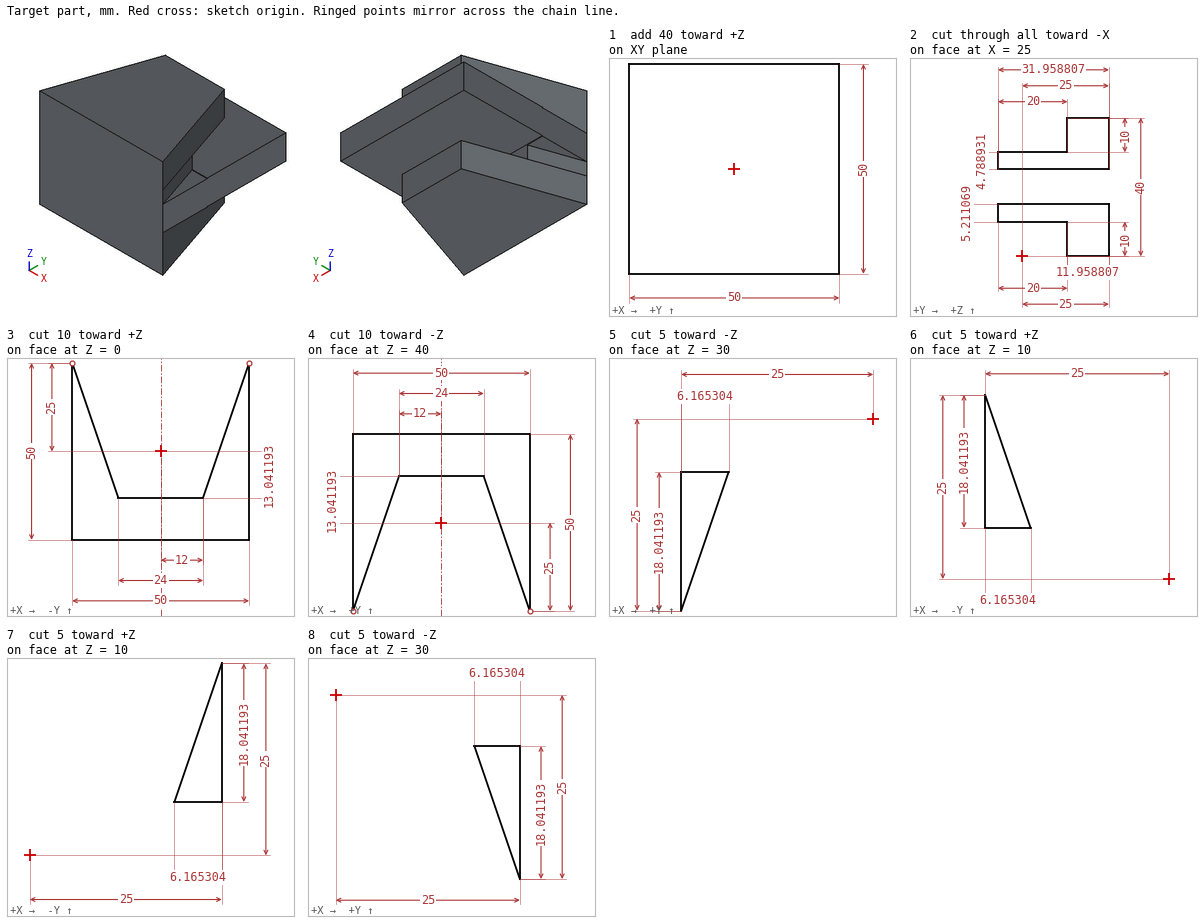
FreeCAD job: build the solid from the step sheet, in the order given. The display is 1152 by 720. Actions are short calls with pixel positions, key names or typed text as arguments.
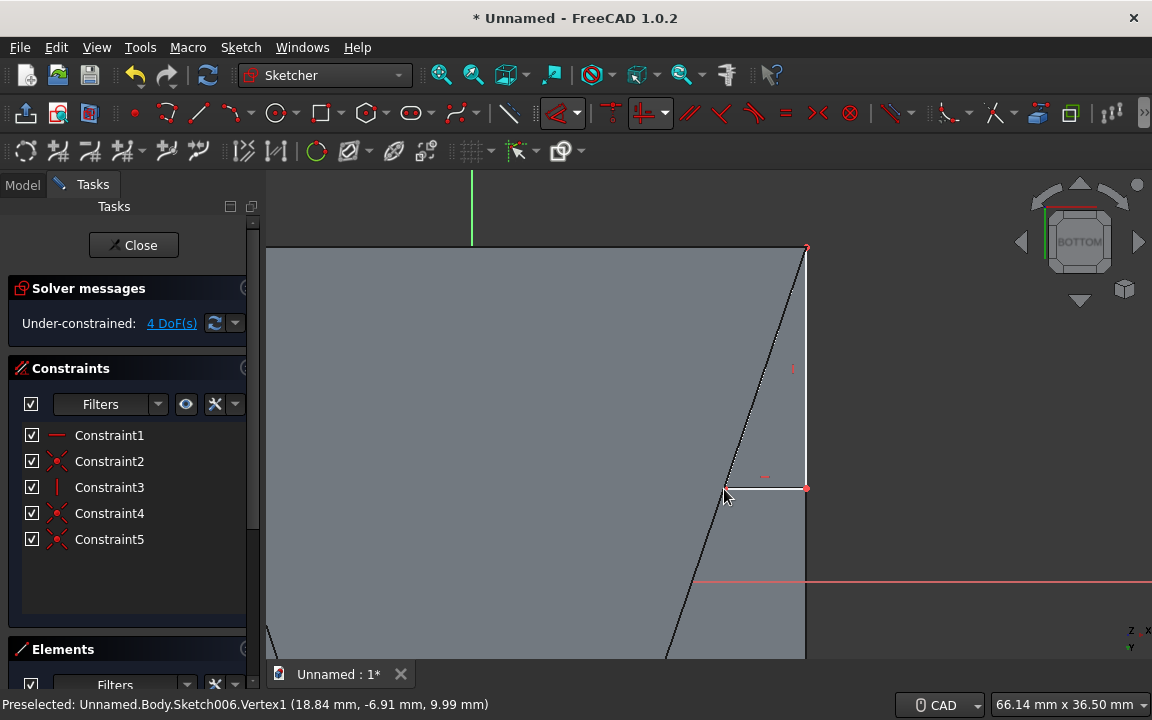
click(806, 489)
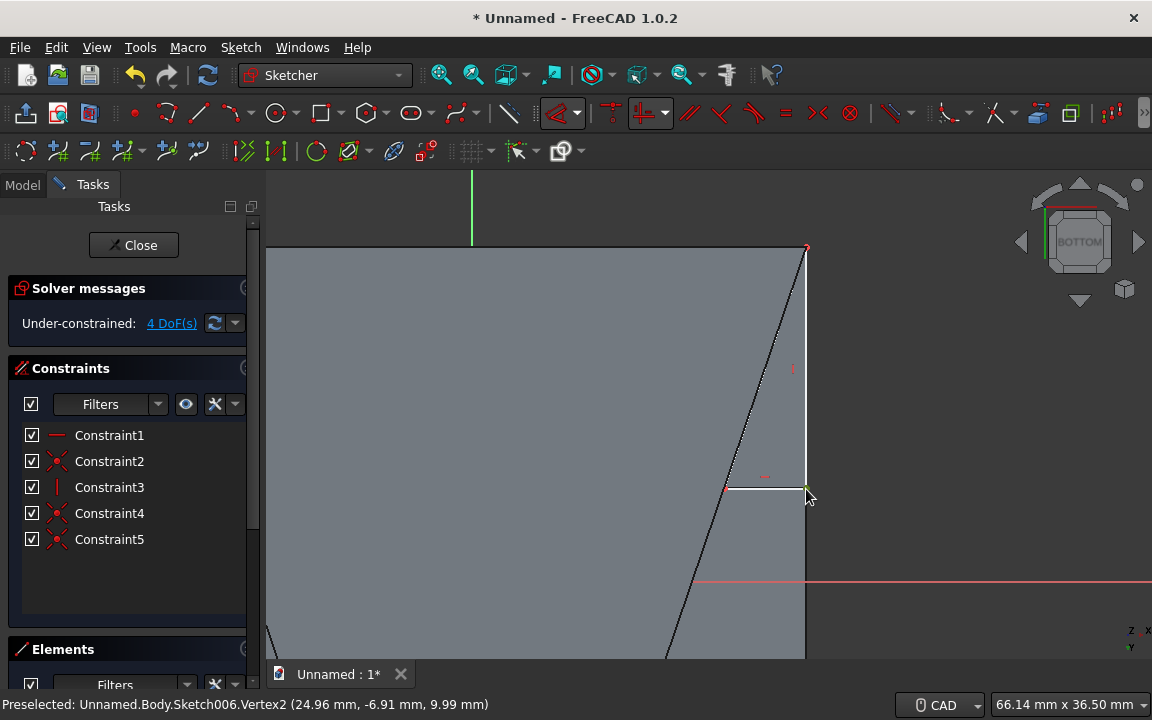
key(l)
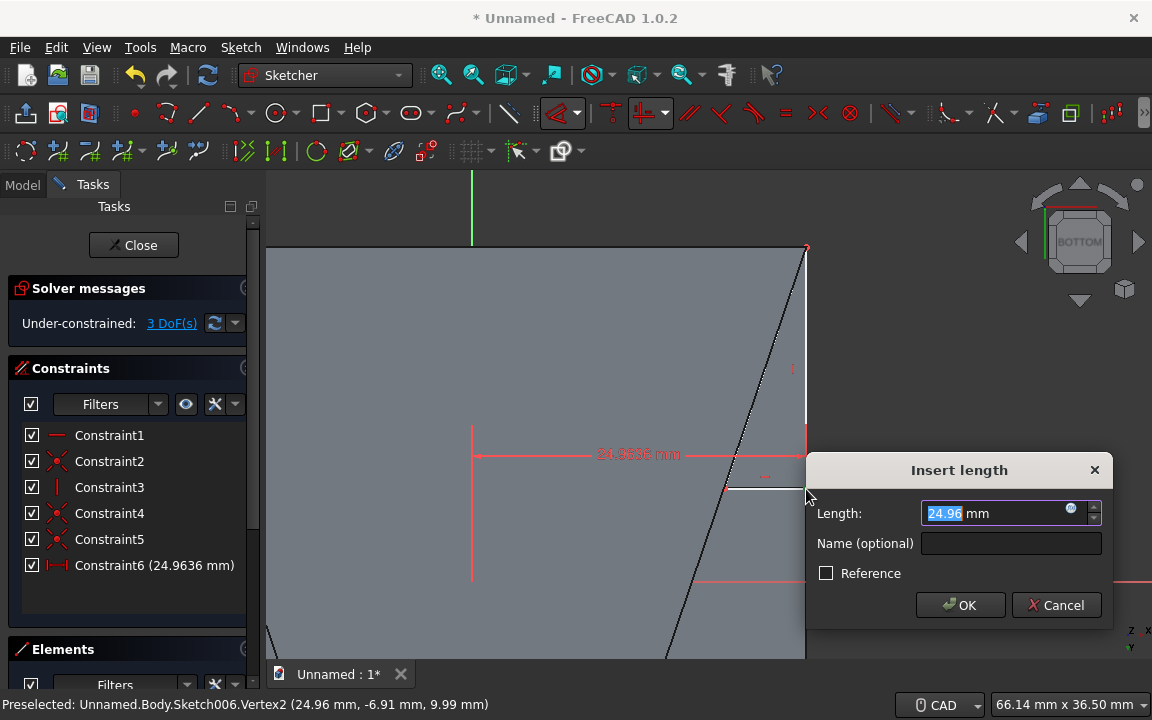
text(25)
key(Return)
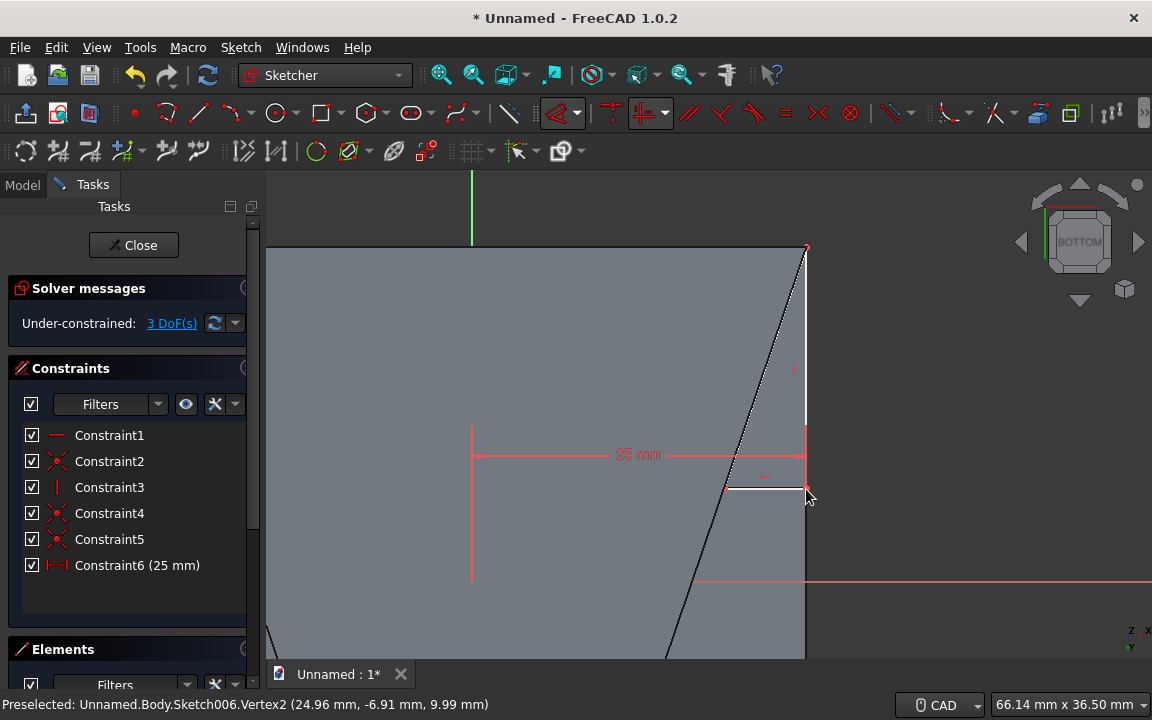
click(806, 248)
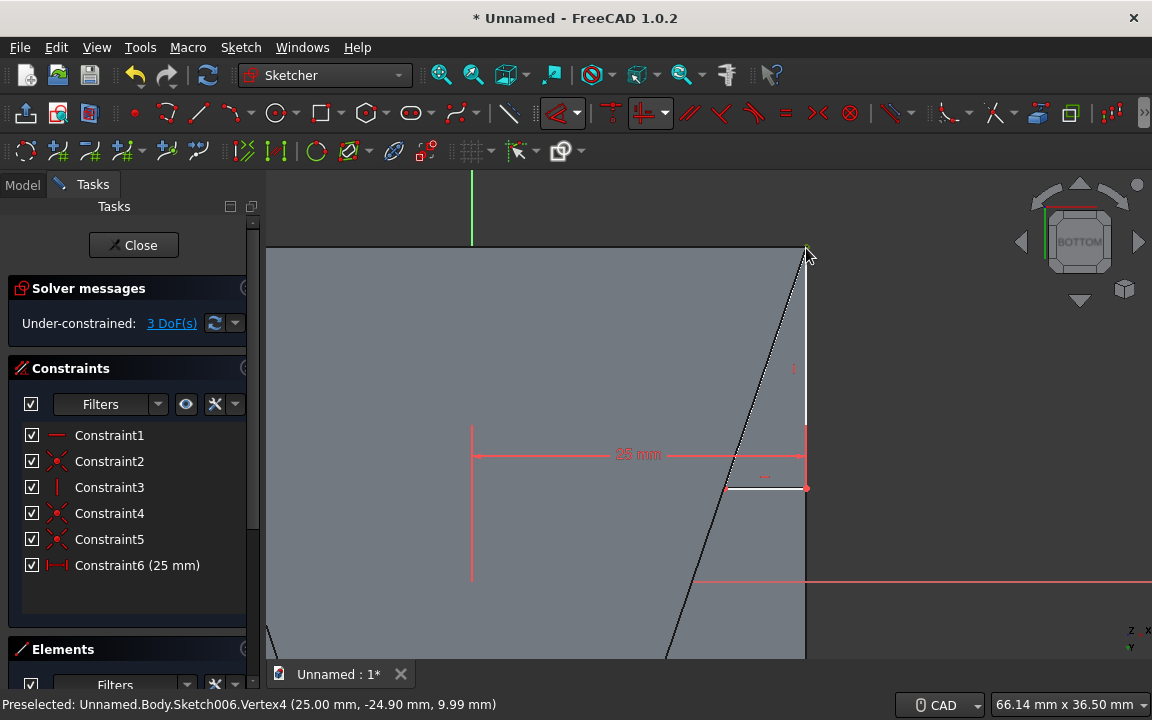
key(i)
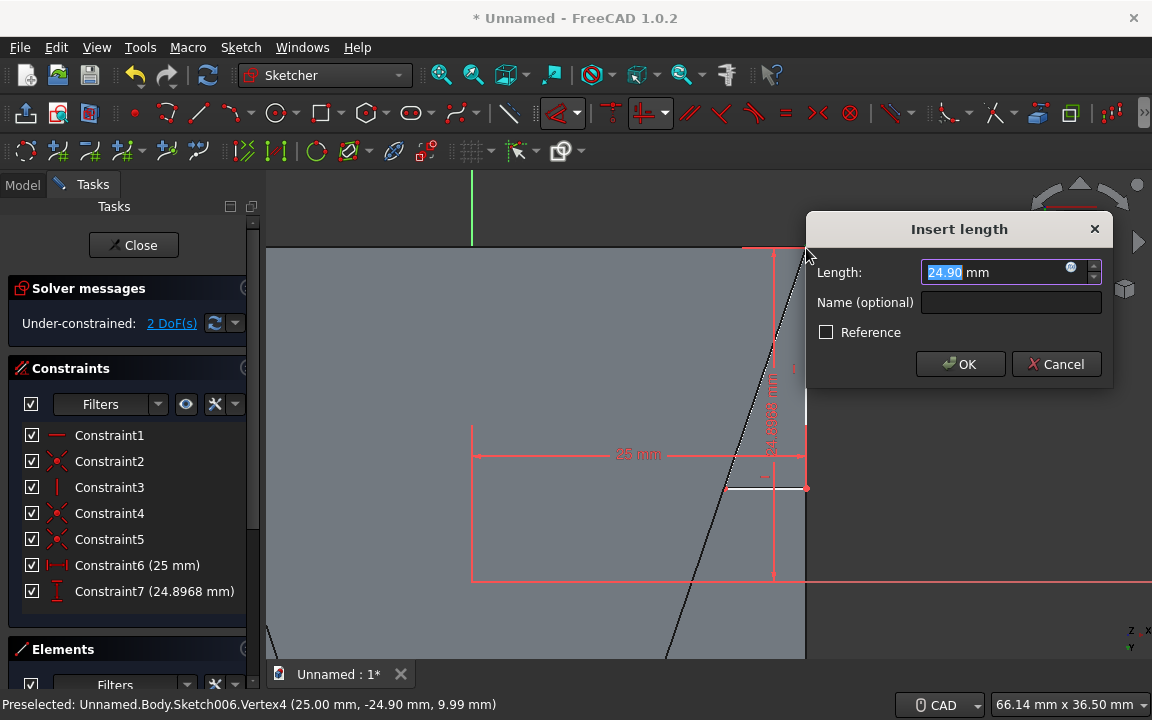
text(25)
key(Return)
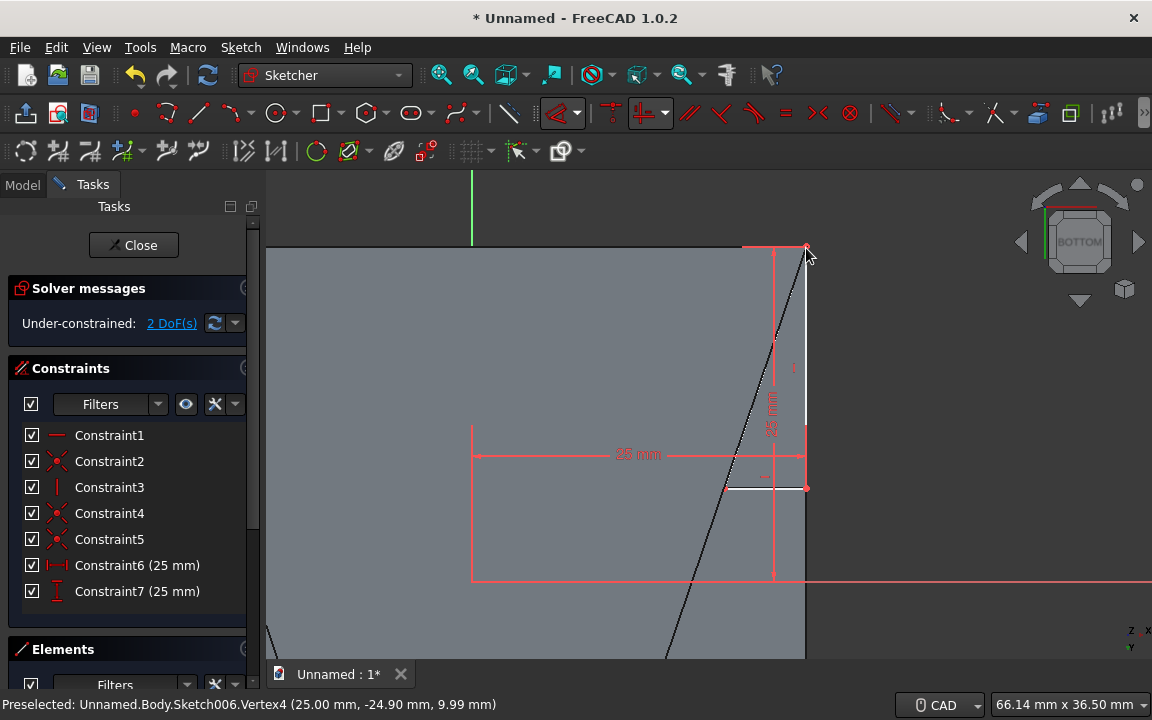
click(749, 489)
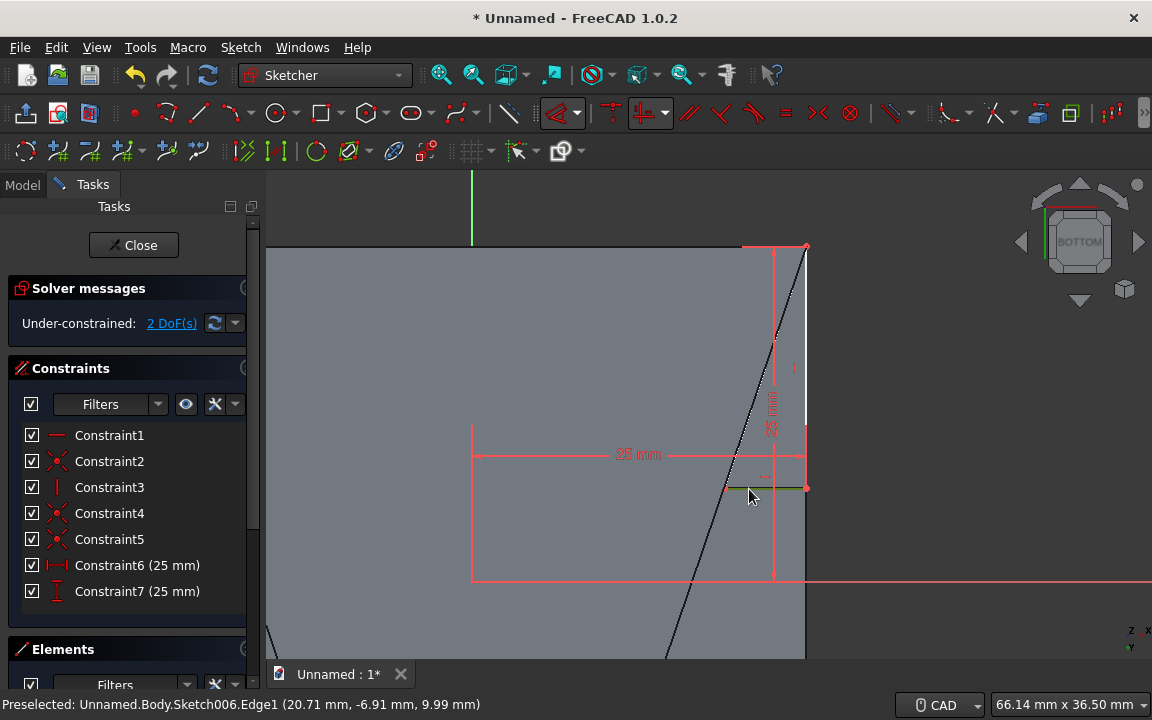
key(l)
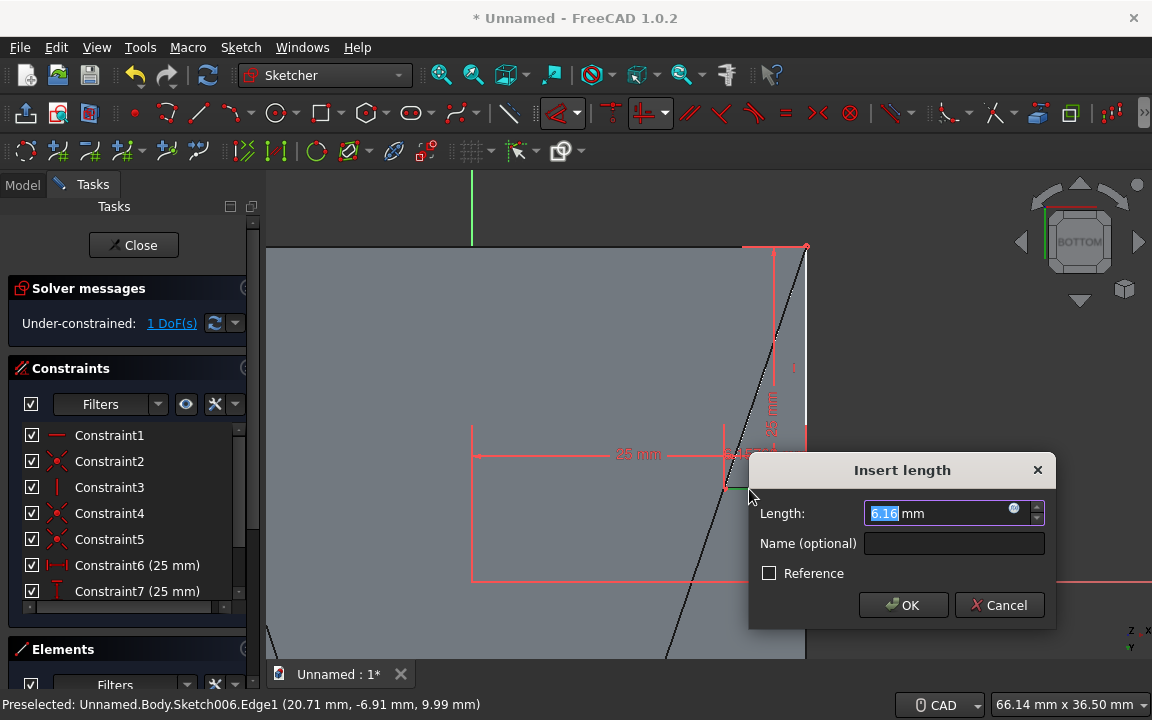
text(6.165304)
key(Return)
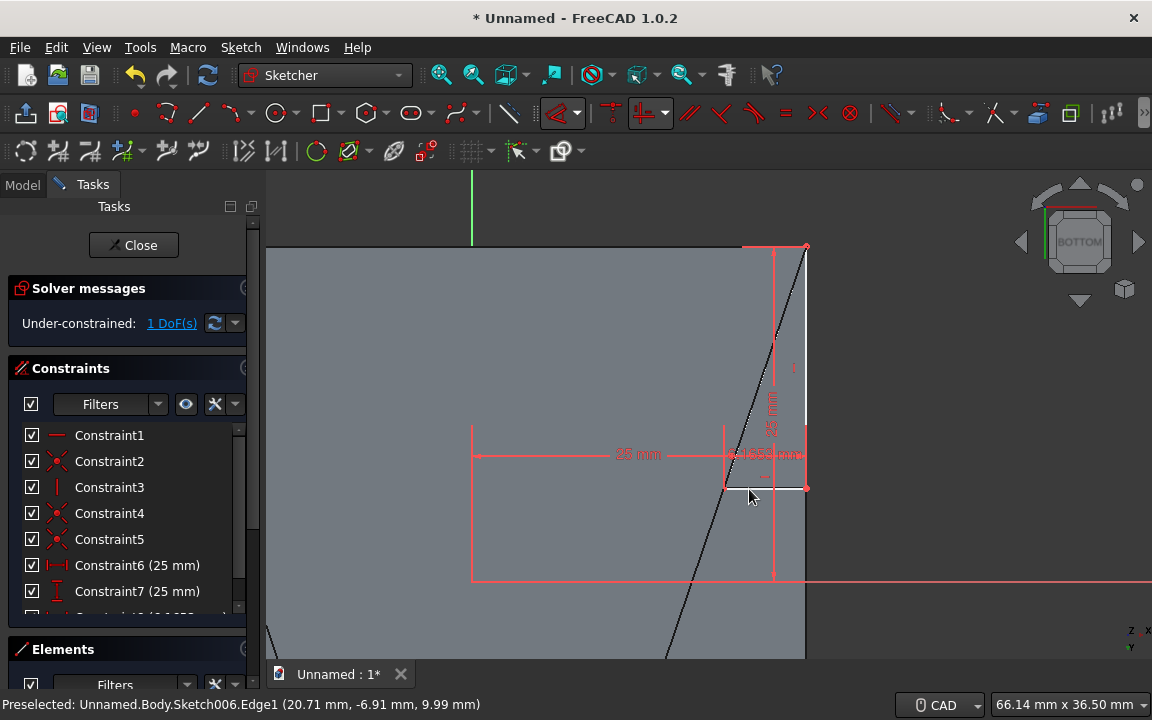
click(806, 416)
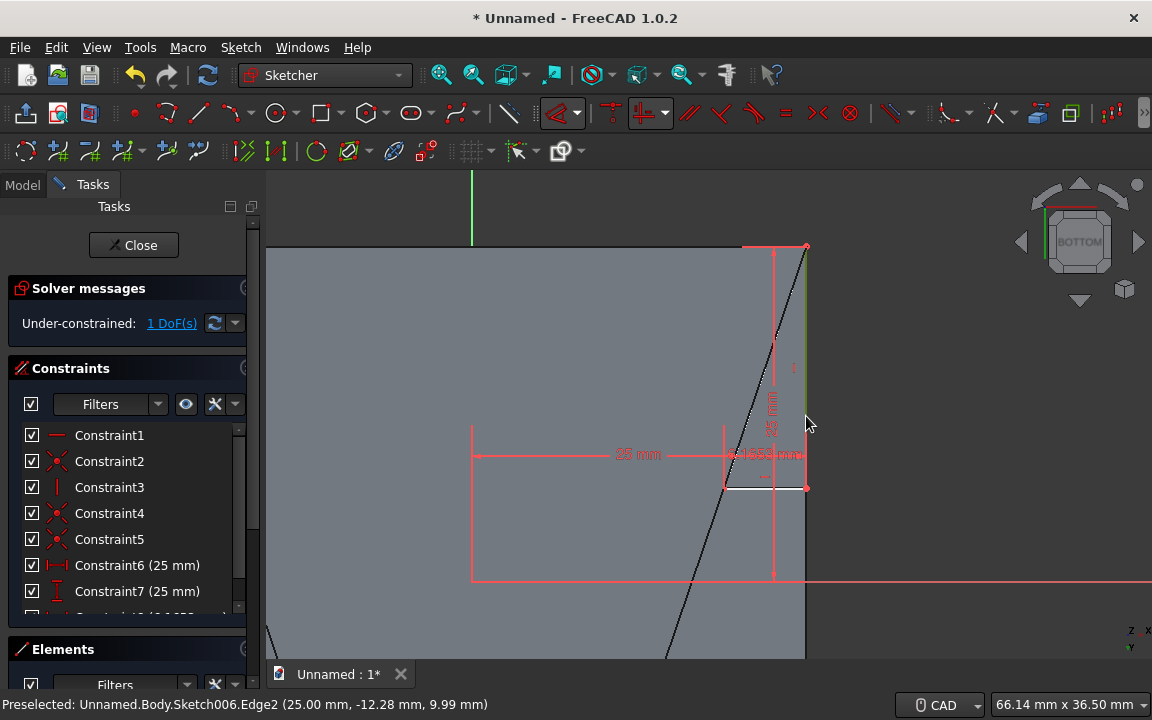
key(i)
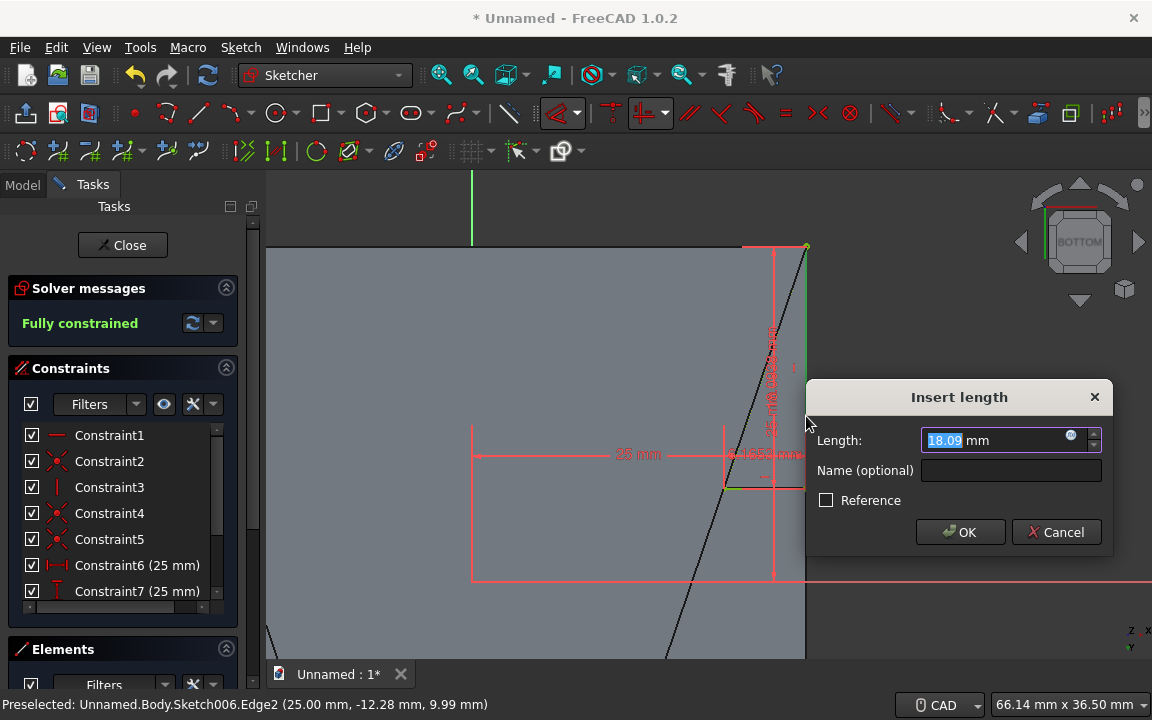
text(18.041193)
key(Return)